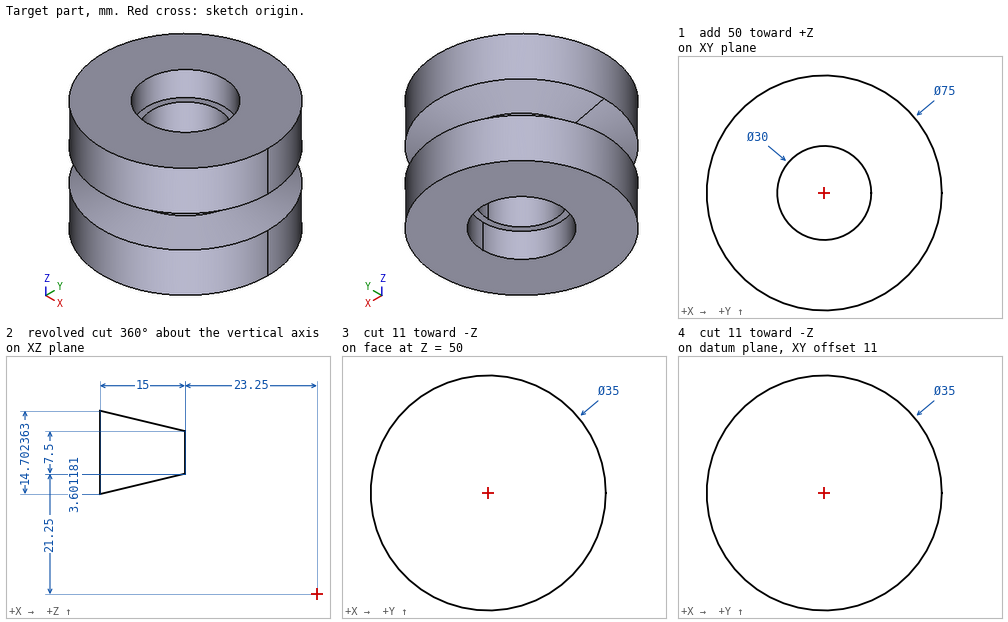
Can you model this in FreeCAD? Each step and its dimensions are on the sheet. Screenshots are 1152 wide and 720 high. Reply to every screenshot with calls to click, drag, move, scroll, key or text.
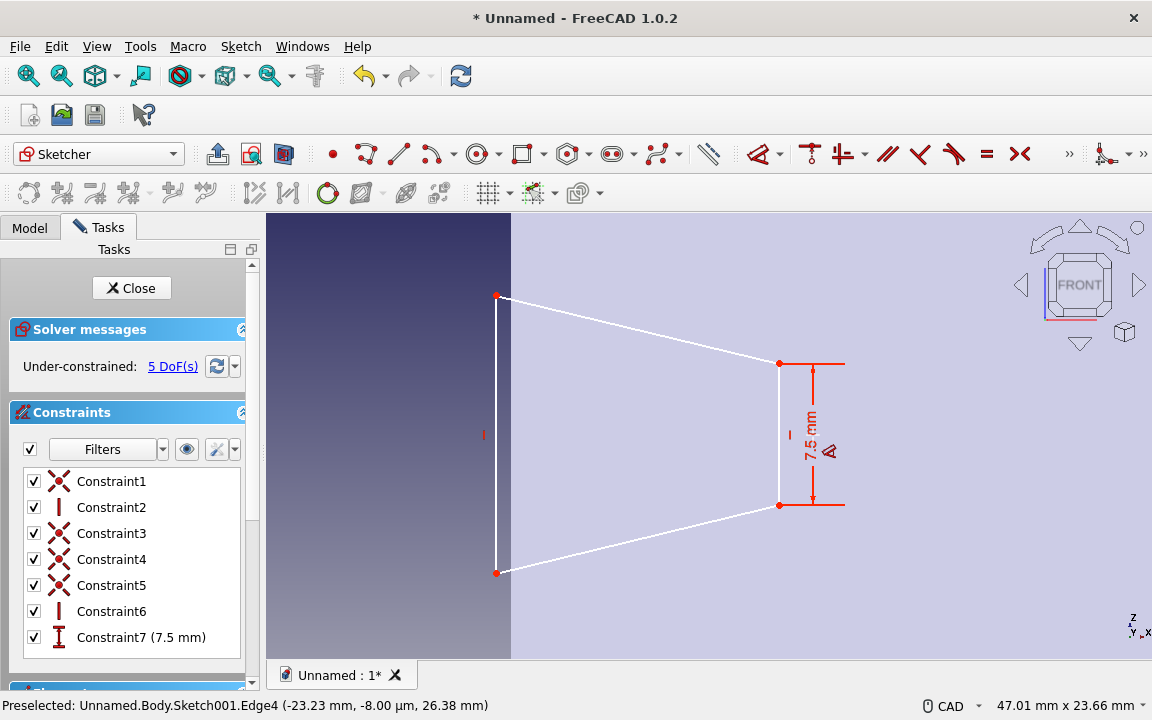
click(694, 526)
click(637, 608)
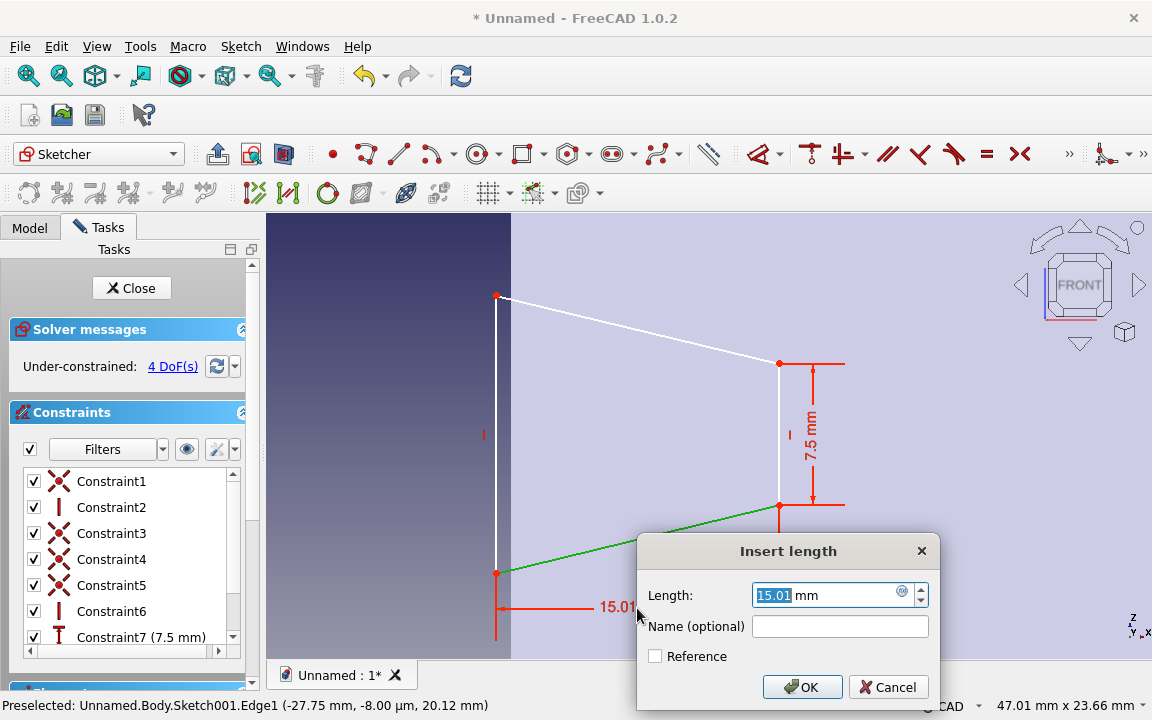
text(15)
key(Return)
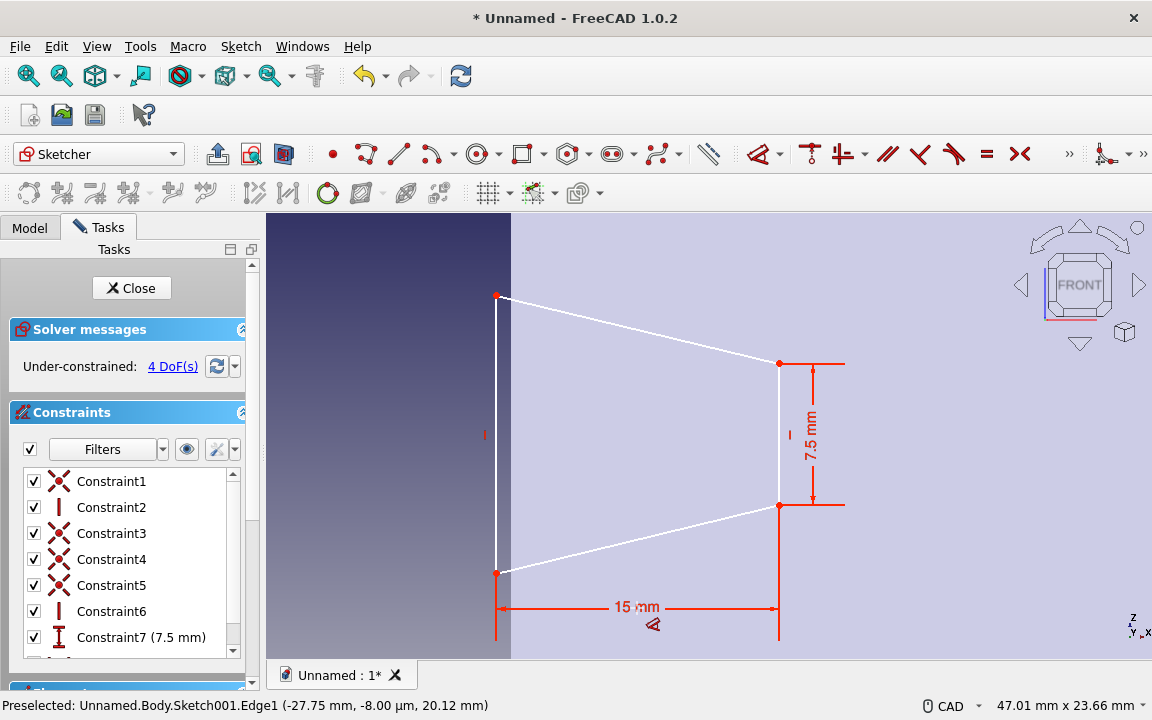
click(779, 505)
click(883, 471)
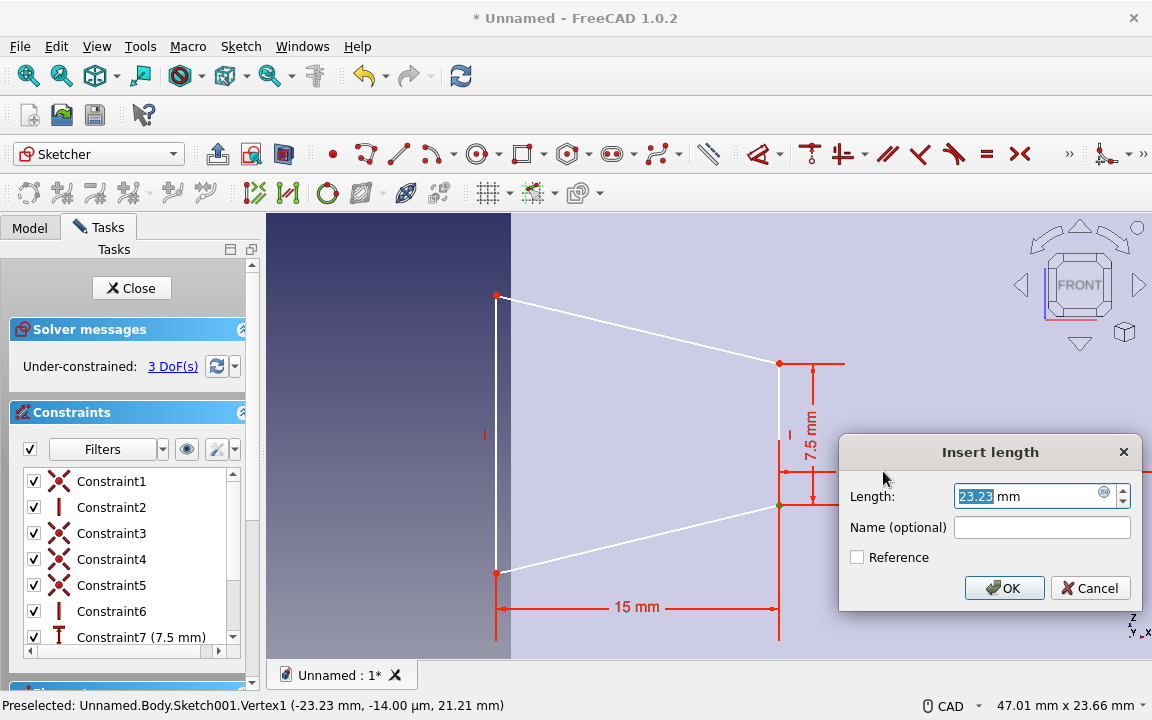
text(23.25)
key(Return)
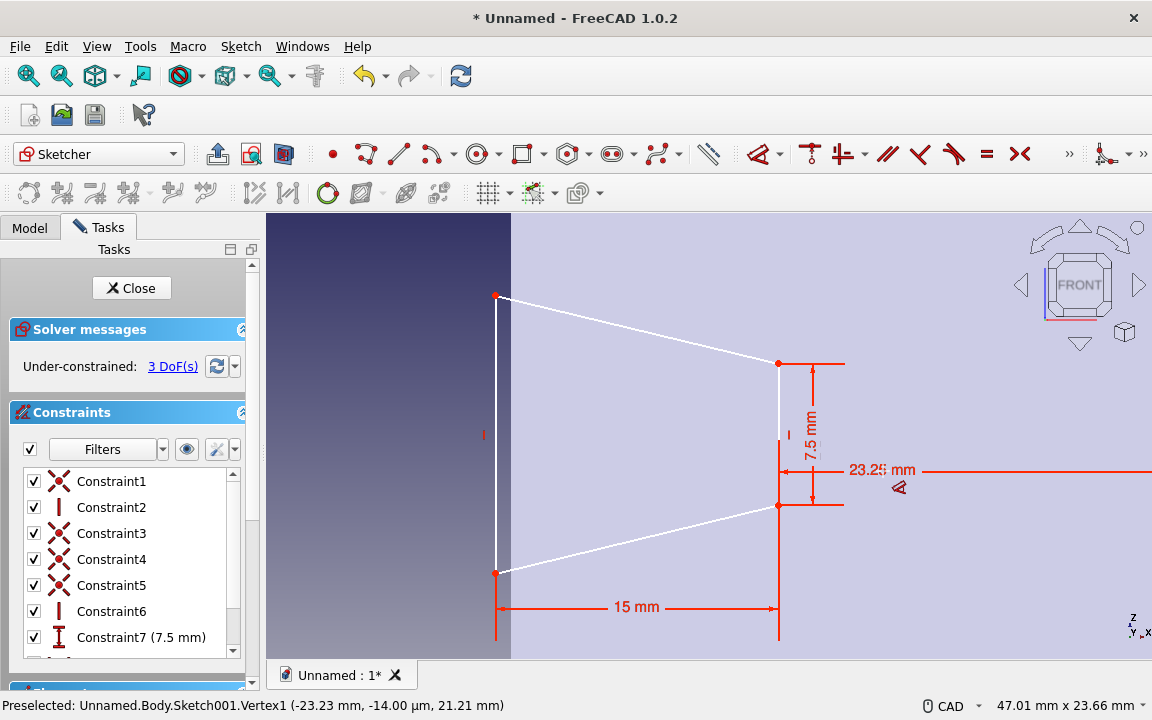
click(779, 505)
click(745, 568)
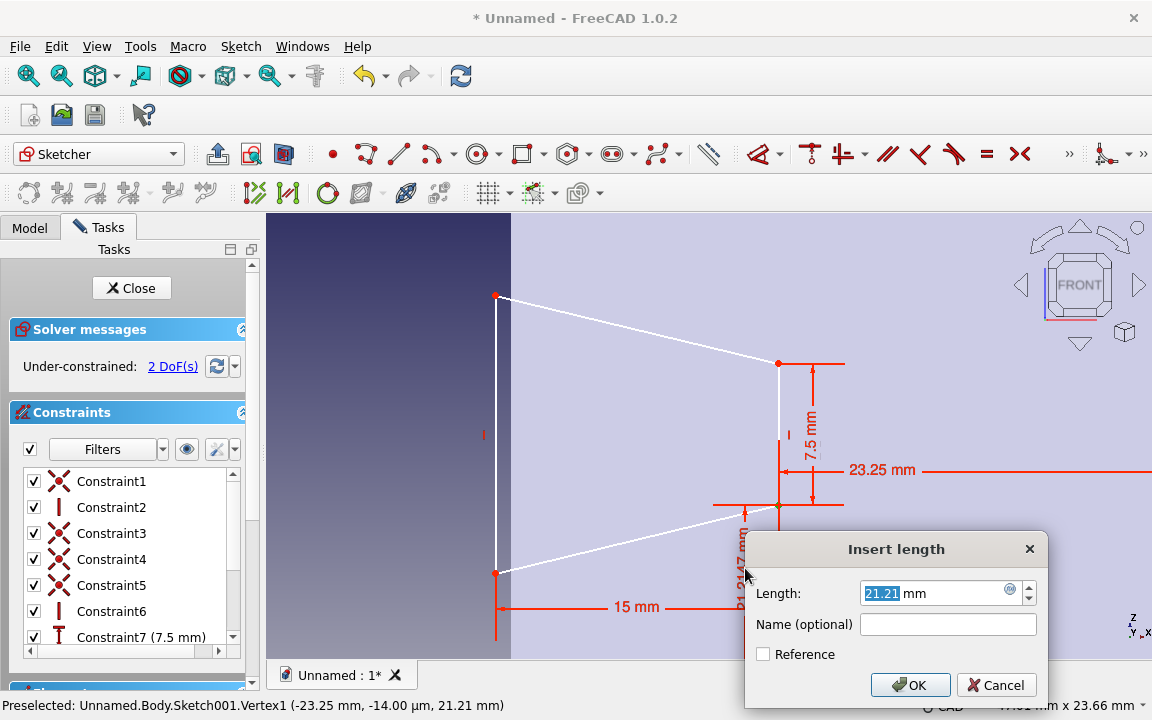
text(21.25)
key(Return)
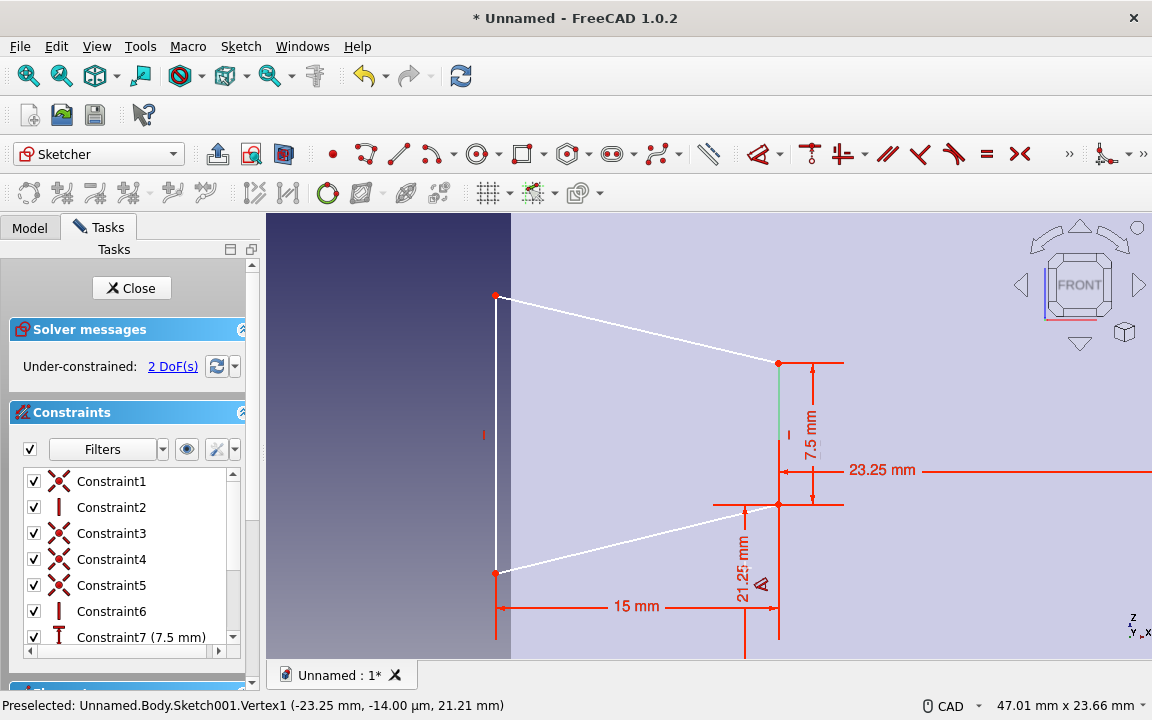
click(496, 491)
click(462, 435)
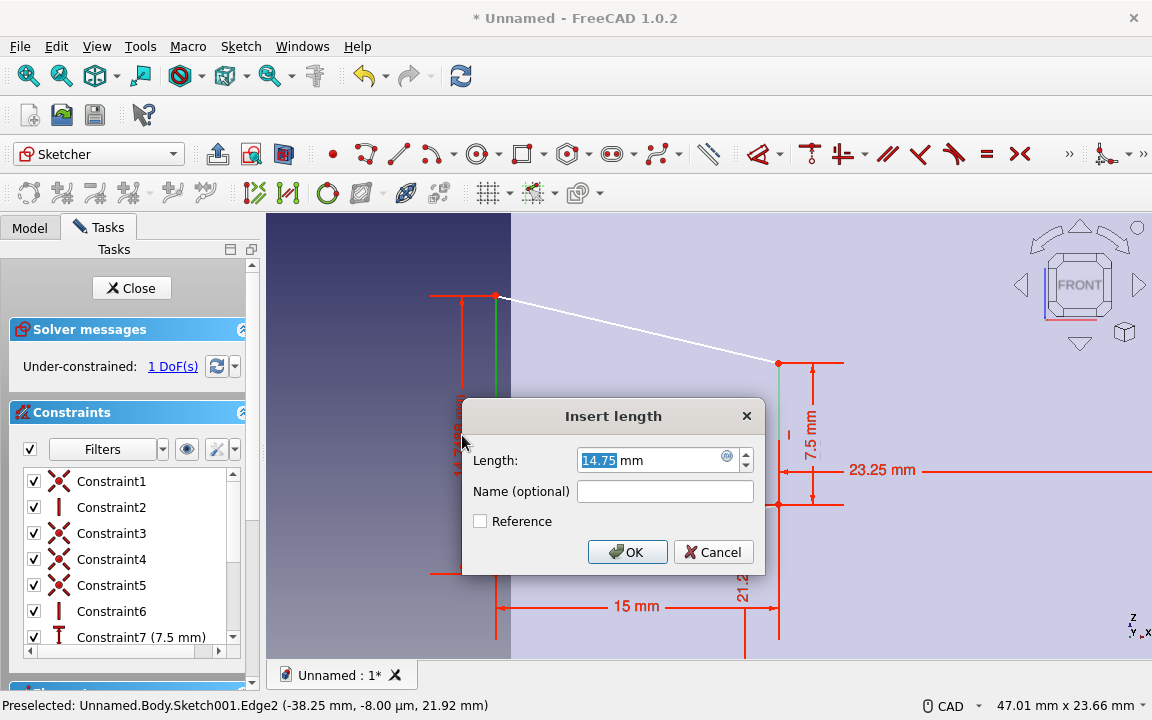
text(14.702363)
key(Return)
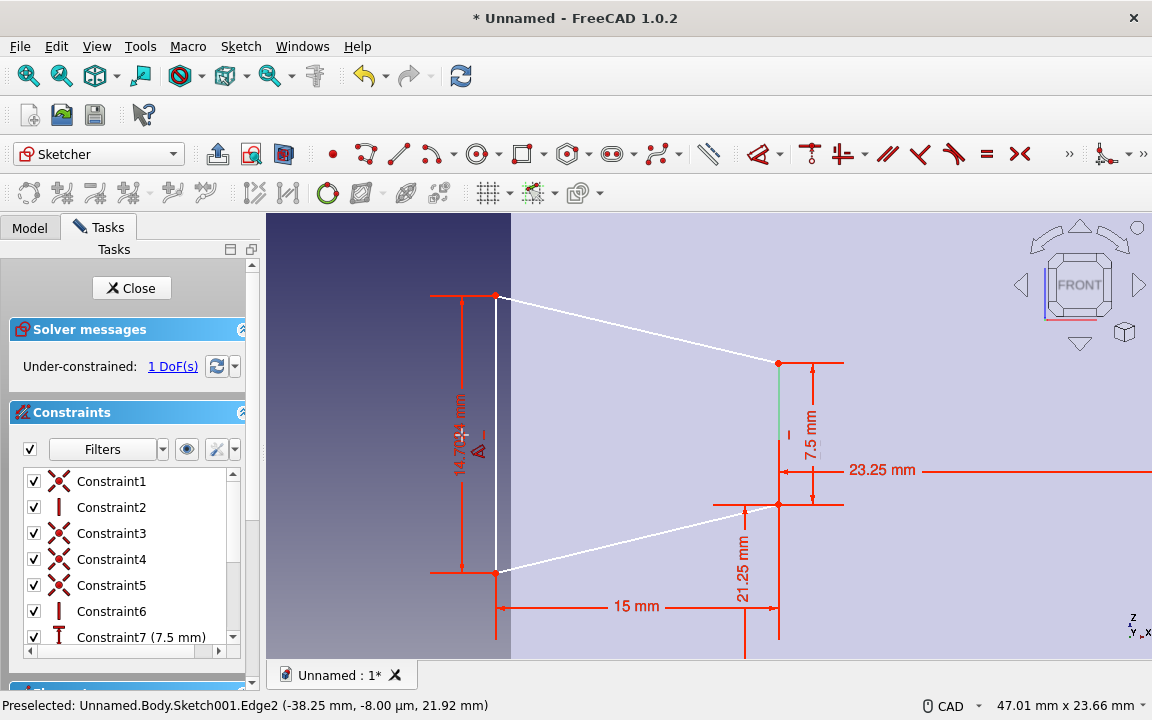
click(694, 525)
click(813, 539)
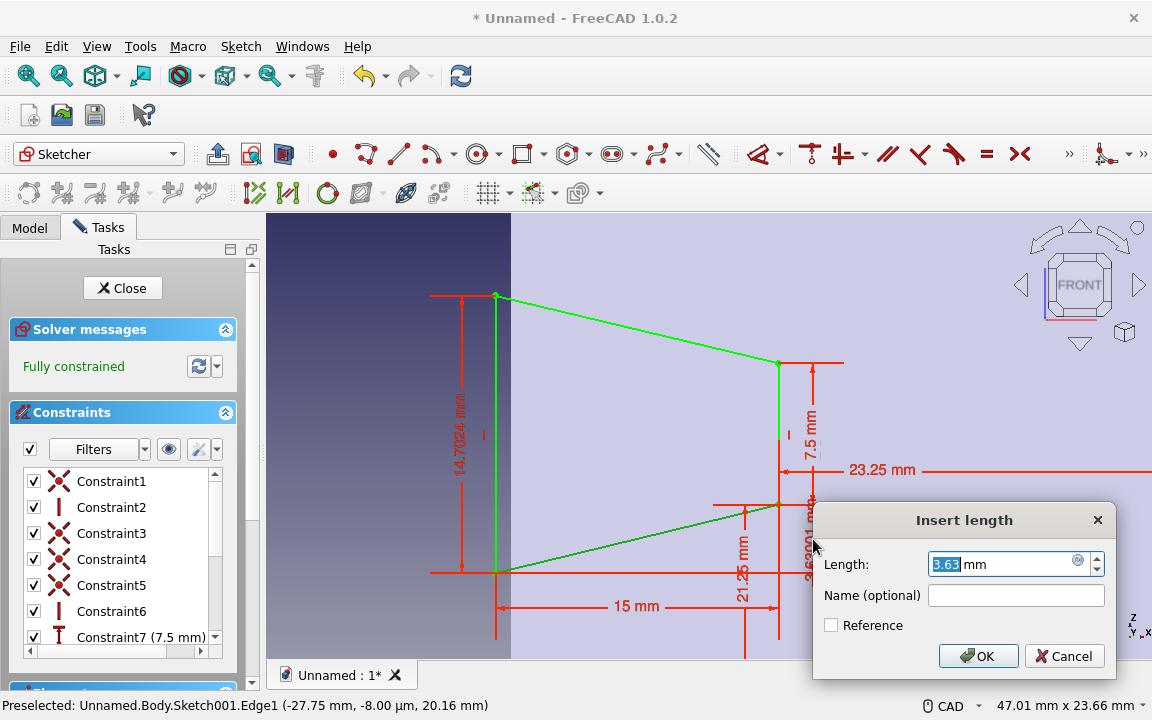
text(3.601181)
key(Return)
key(Escape)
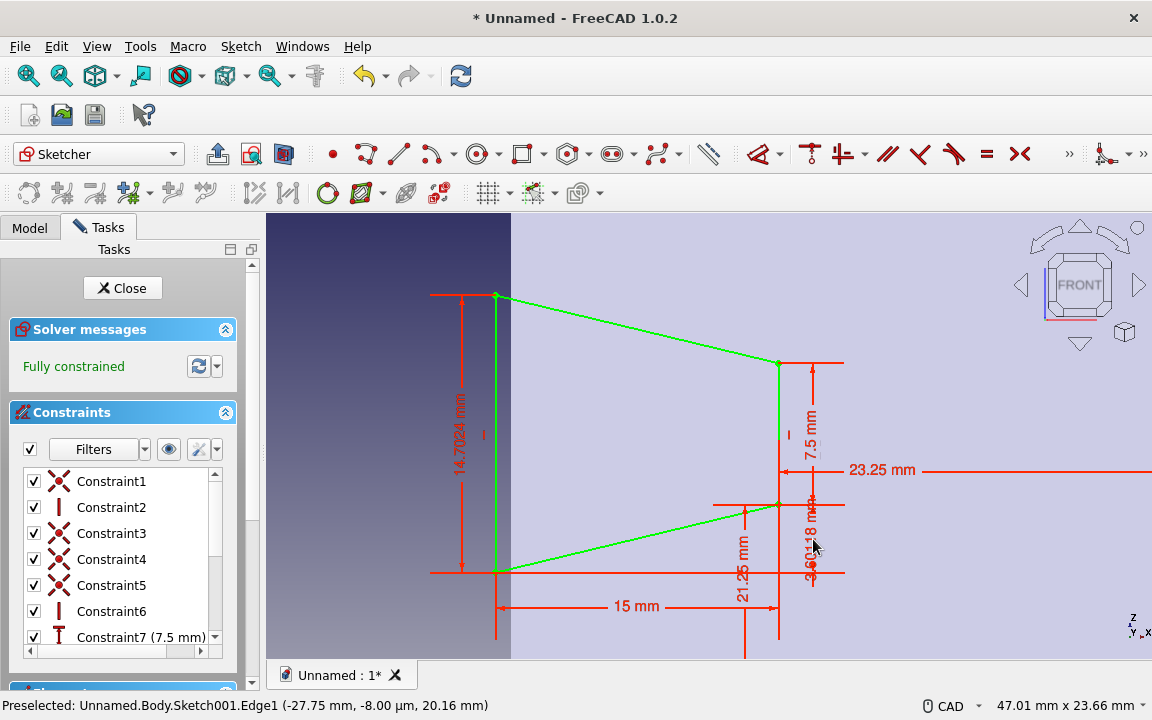
click(123, 288)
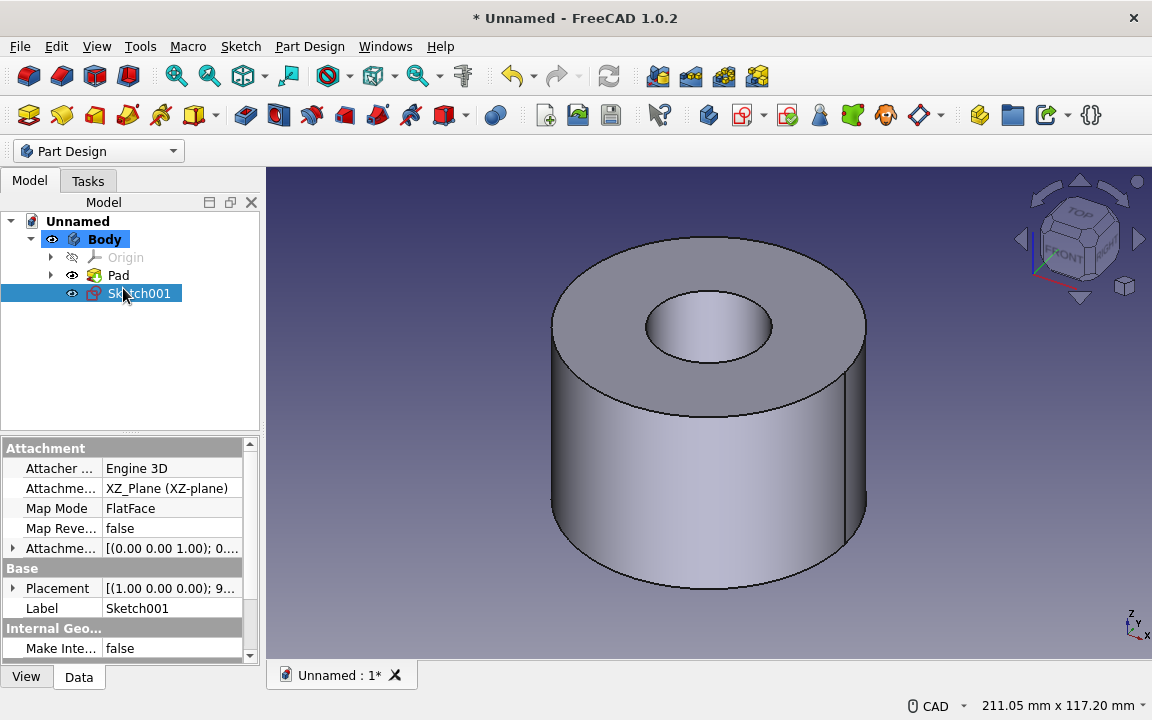
click(312, 116)